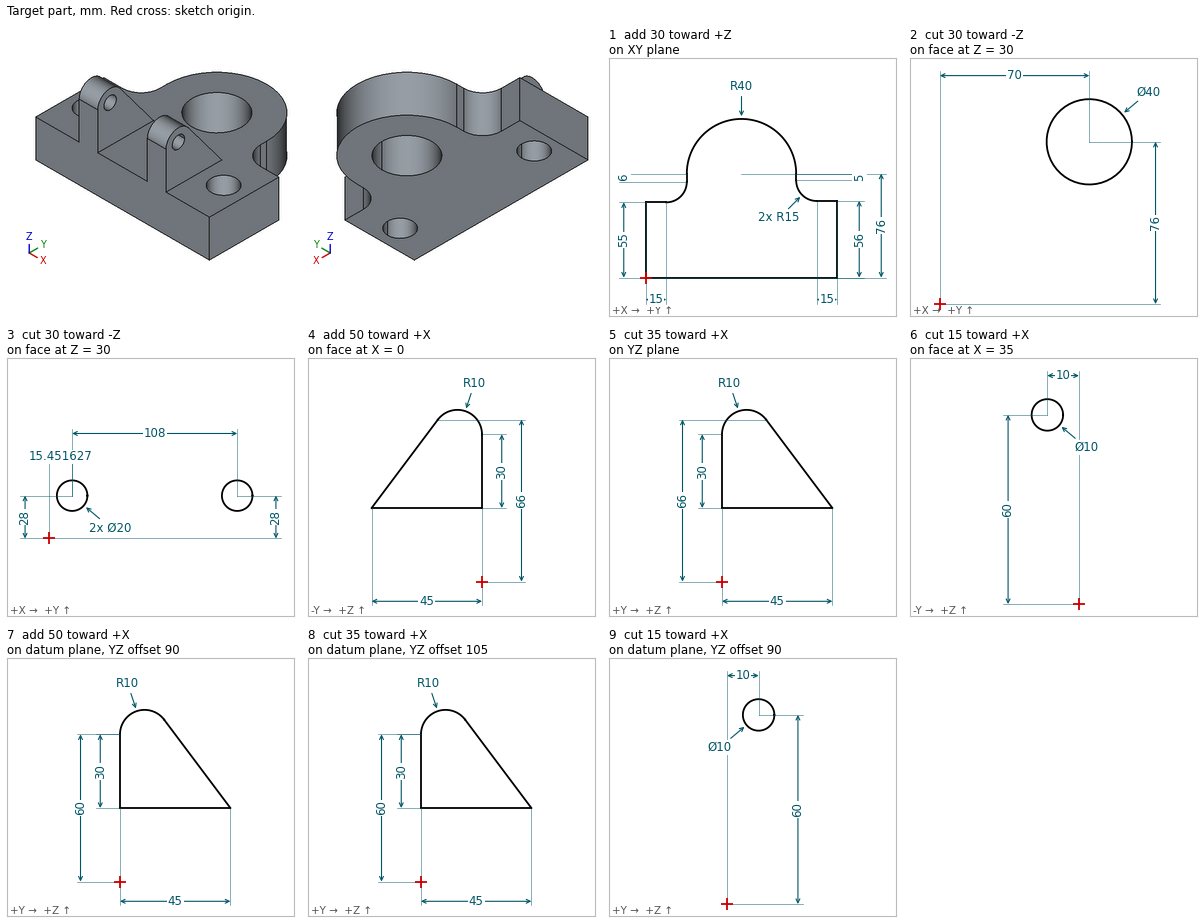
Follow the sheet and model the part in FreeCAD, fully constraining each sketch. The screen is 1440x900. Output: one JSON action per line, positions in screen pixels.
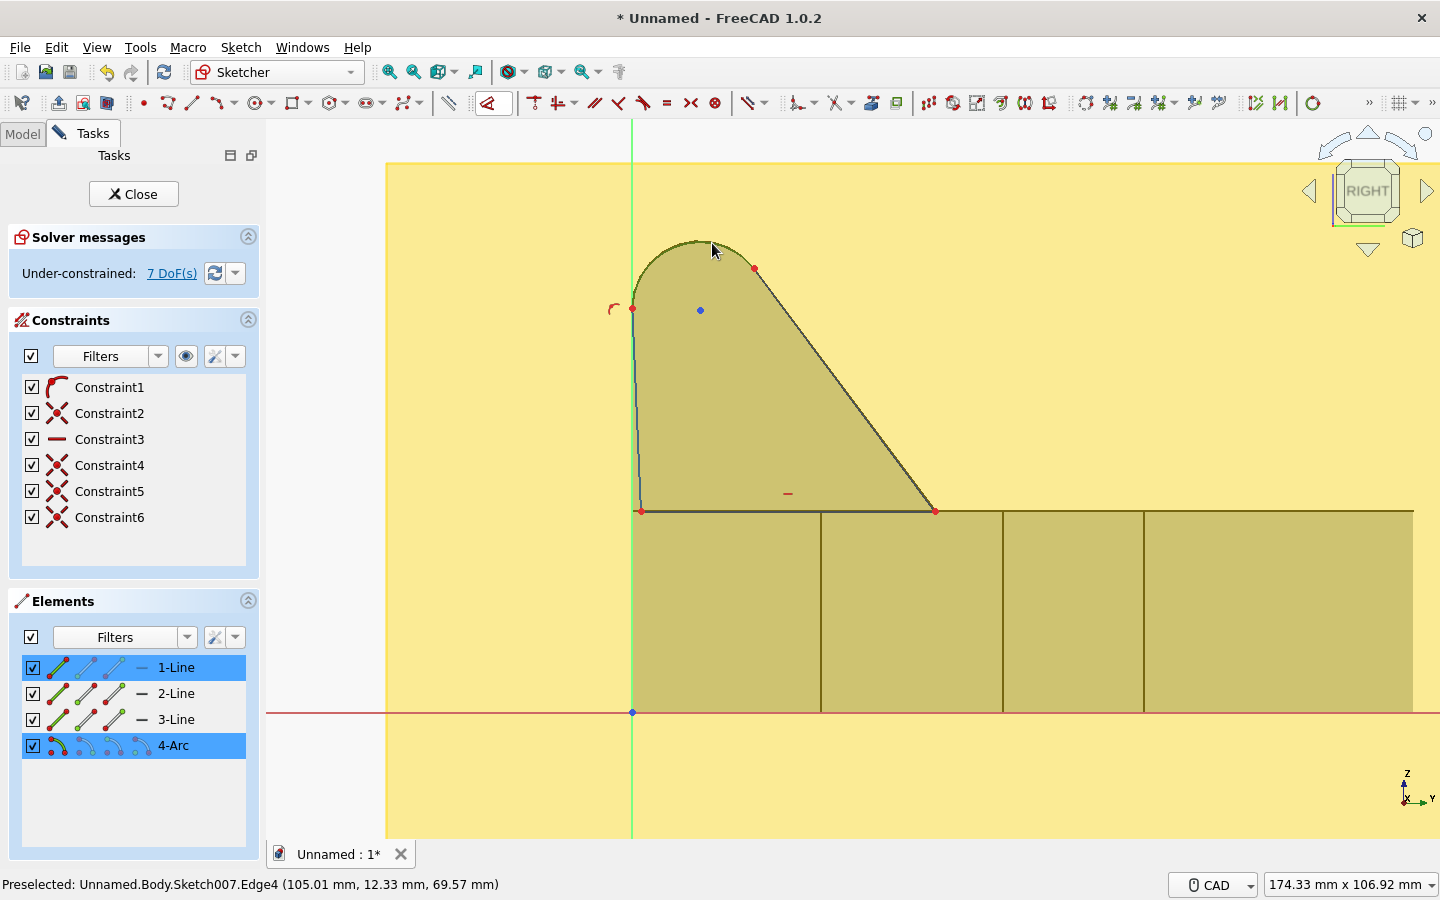
{"action": "key", "text": "t"}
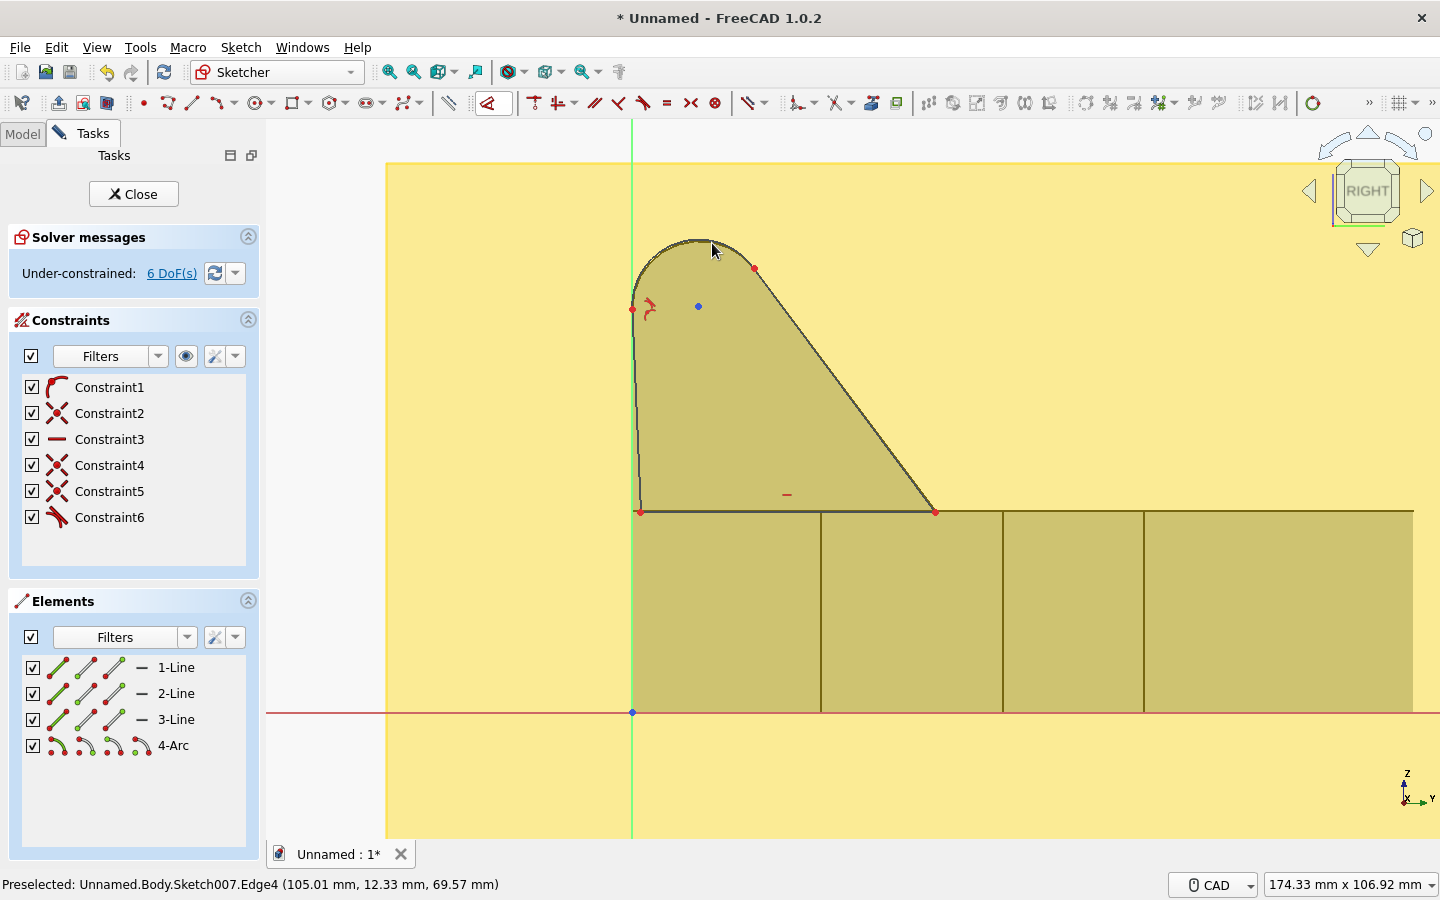
{"action": "left_click", "coordinate": [881, 439]}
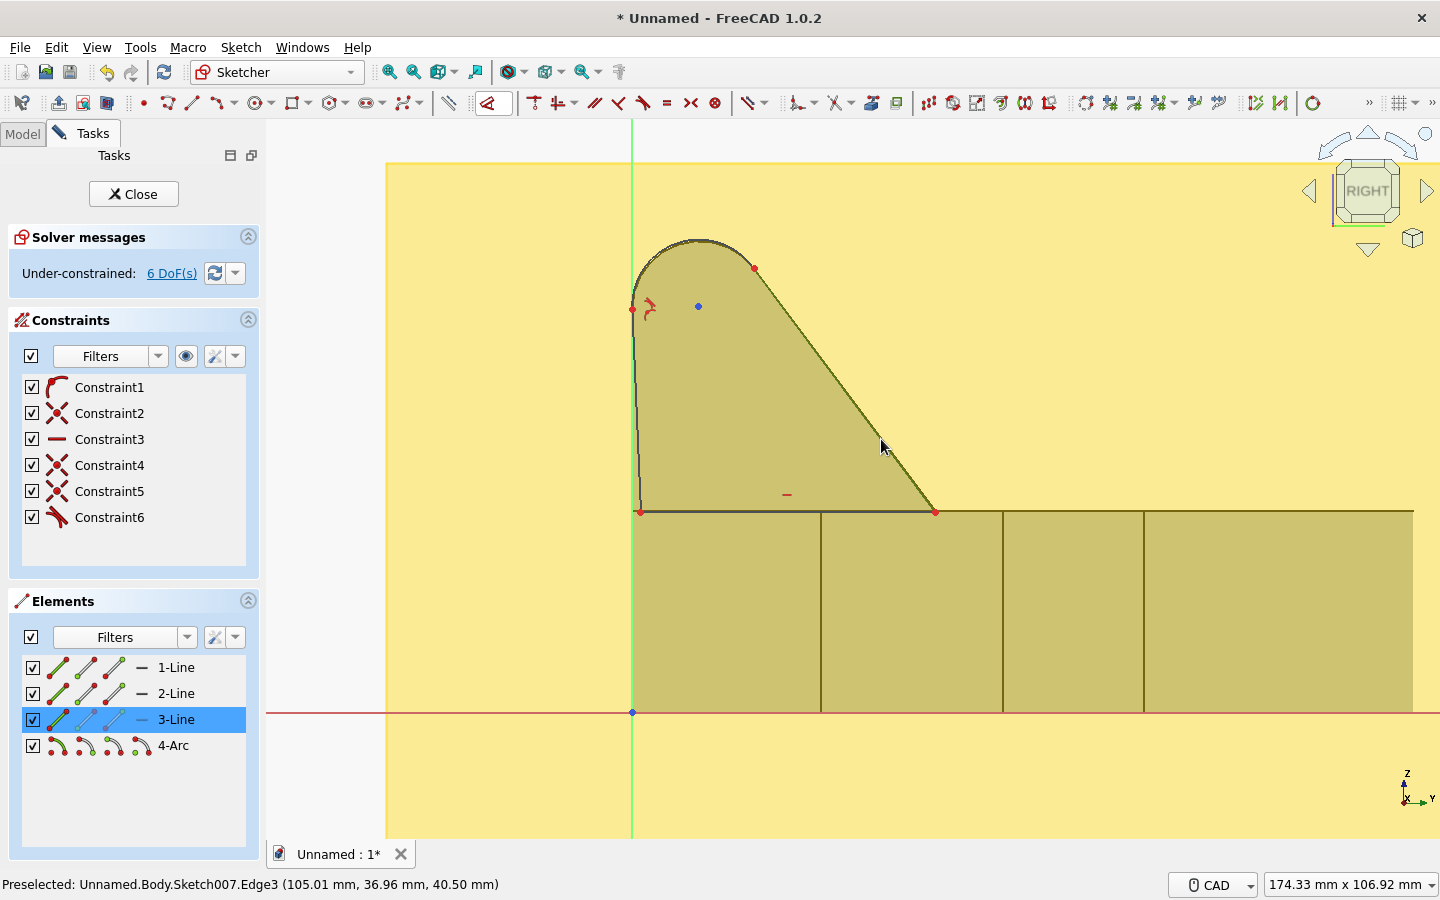
{"action": "left_click", "coordinate": [712, 241]}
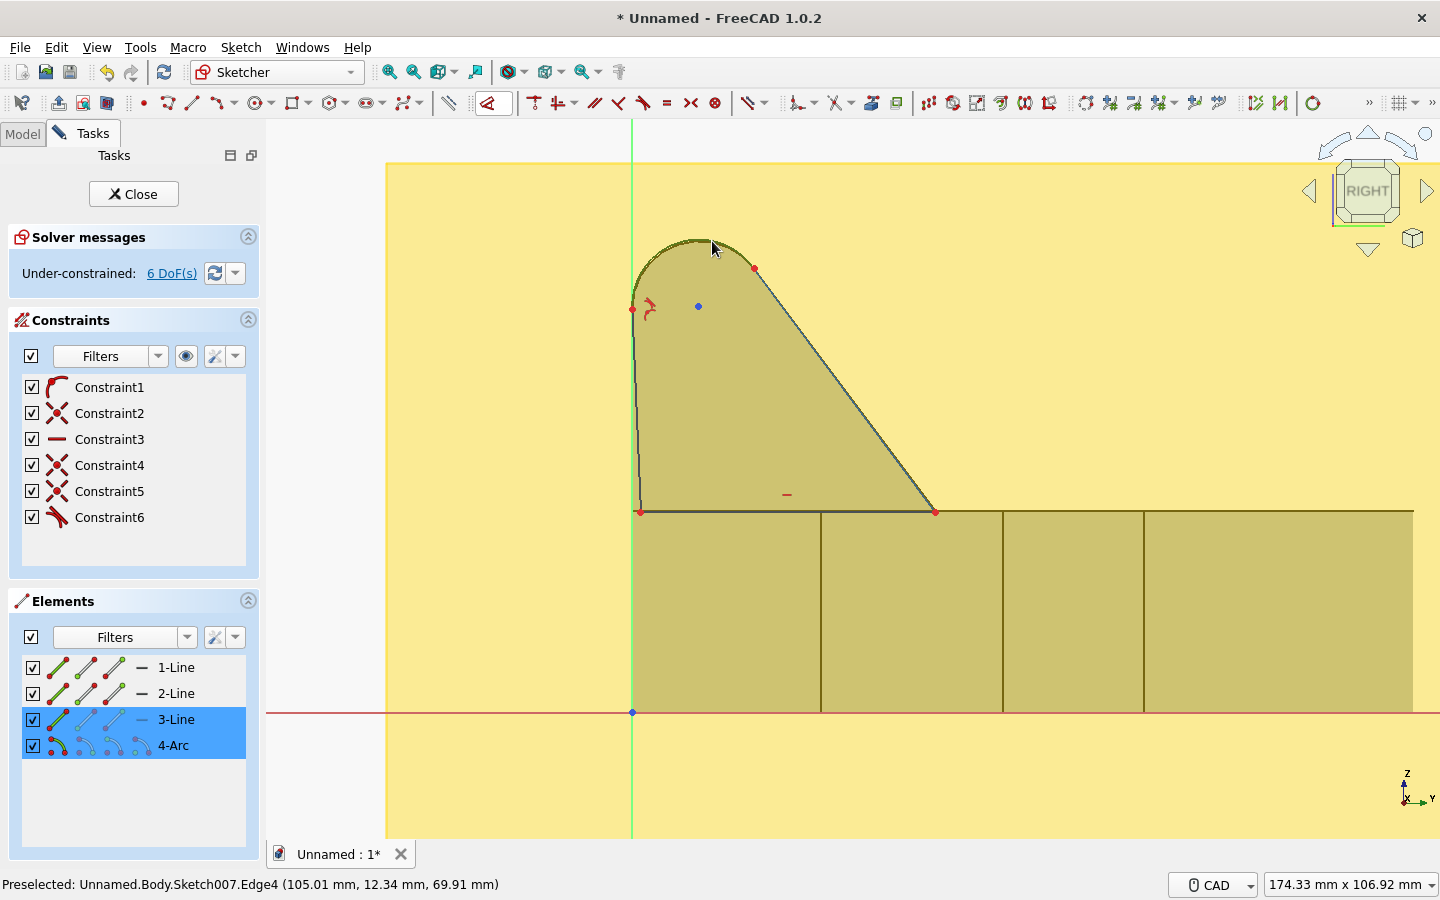
{"action": "left_click", "coordinate": [644, 104]}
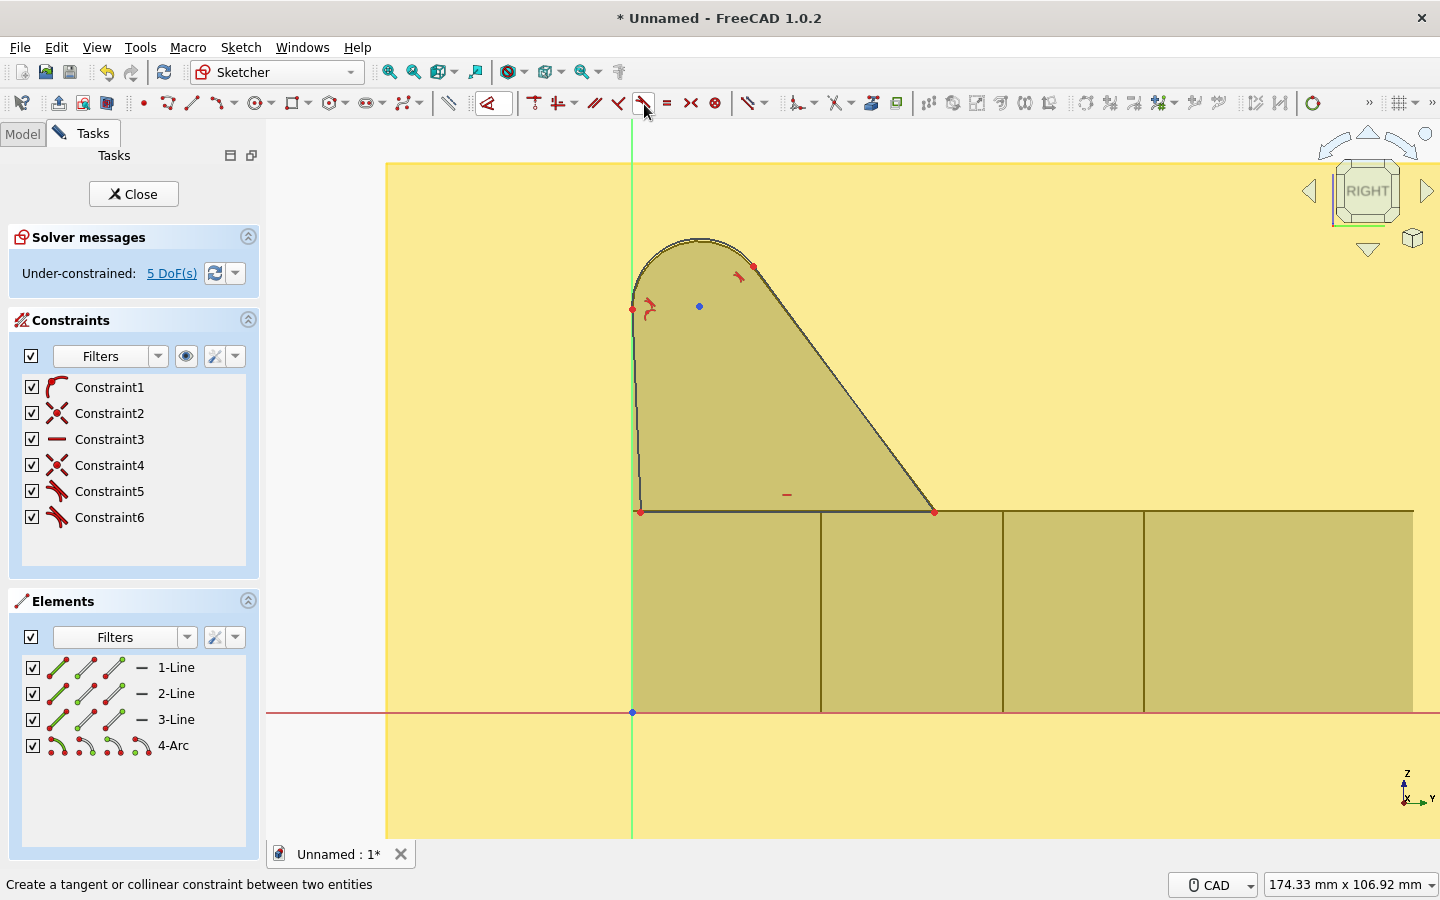
{"action": "left_click", "coordinate": [635, 370]}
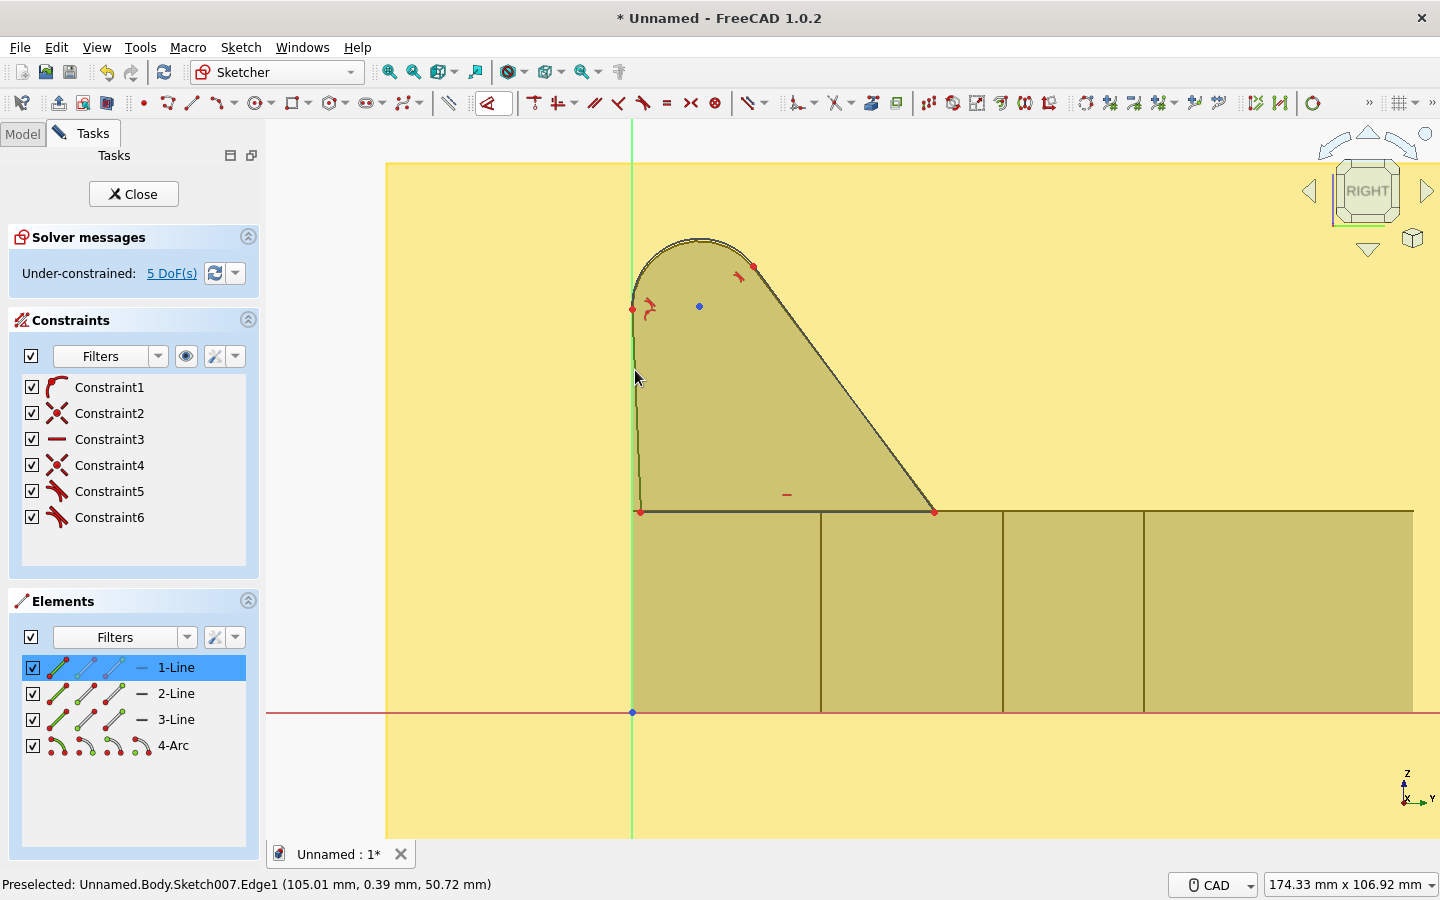
{"action": "key", "text": "v"}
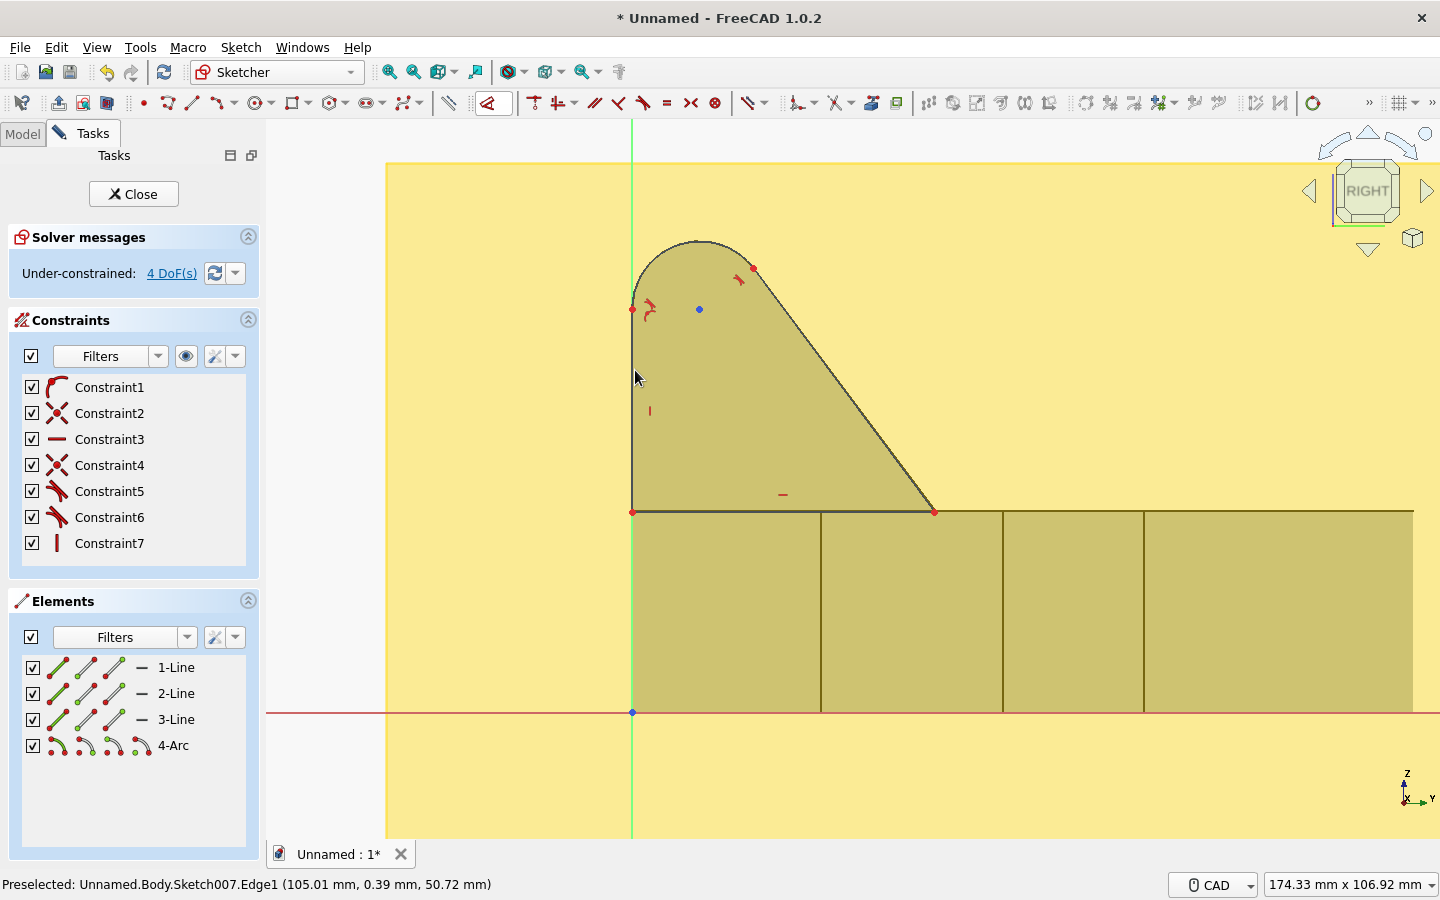
{"action": "left_click", "coordinate": [712, 243]}